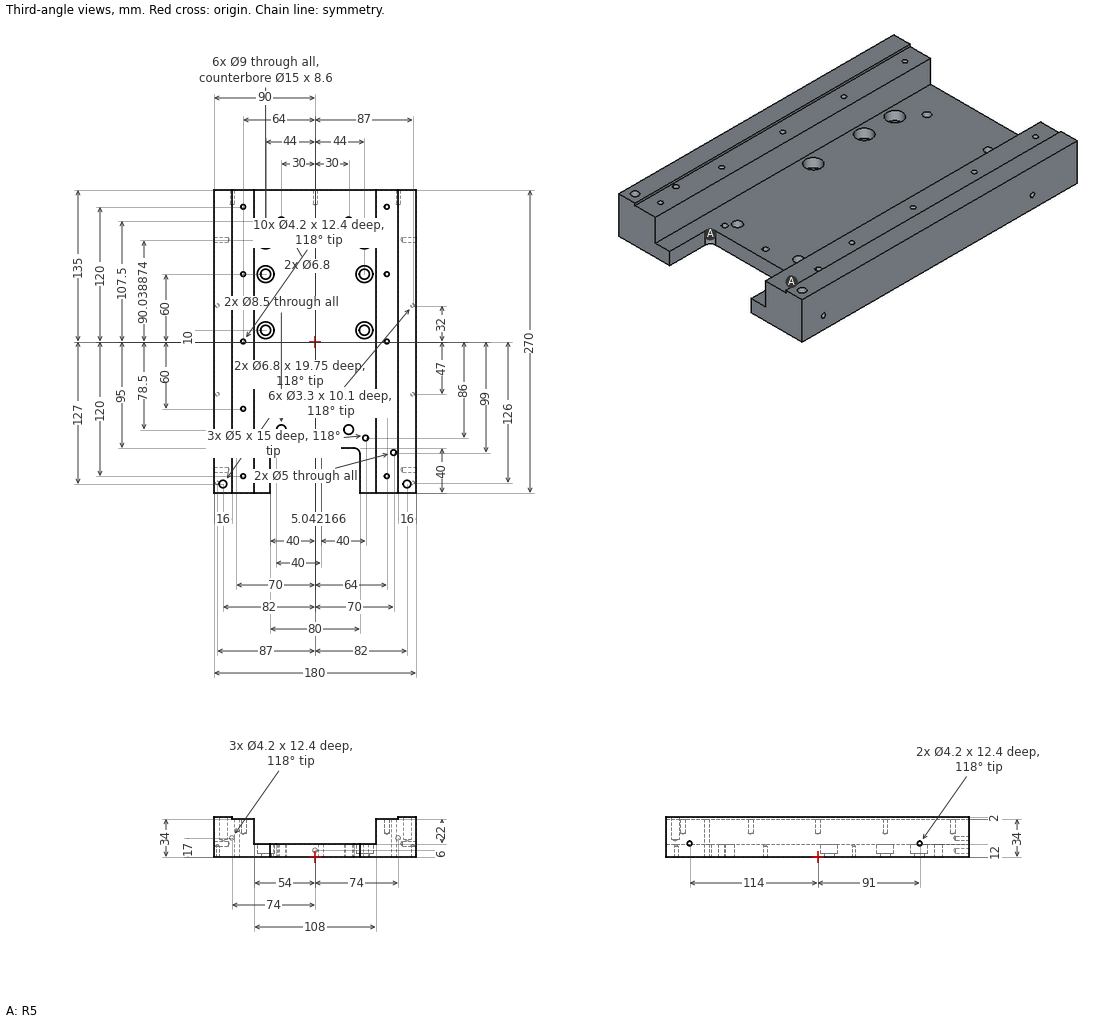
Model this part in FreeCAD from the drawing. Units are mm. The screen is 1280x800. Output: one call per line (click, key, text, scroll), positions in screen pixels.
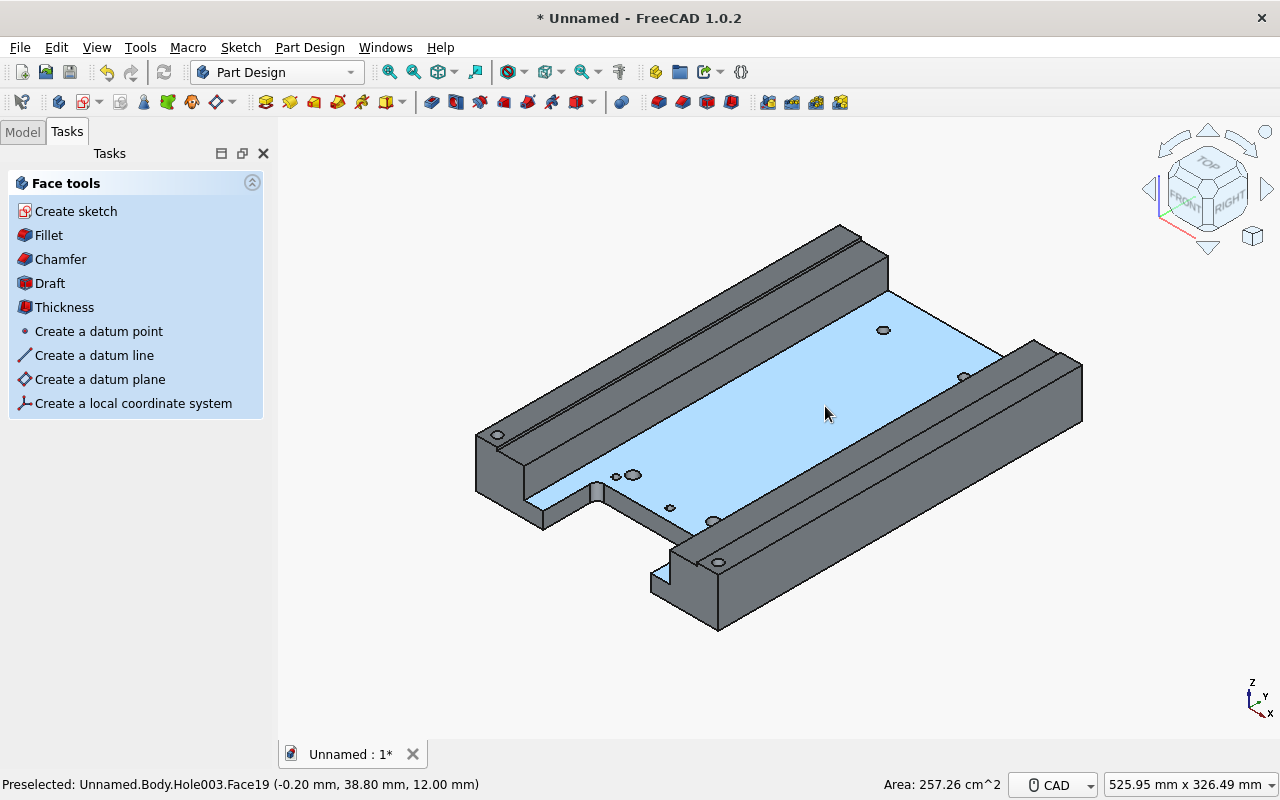
click(84, 102)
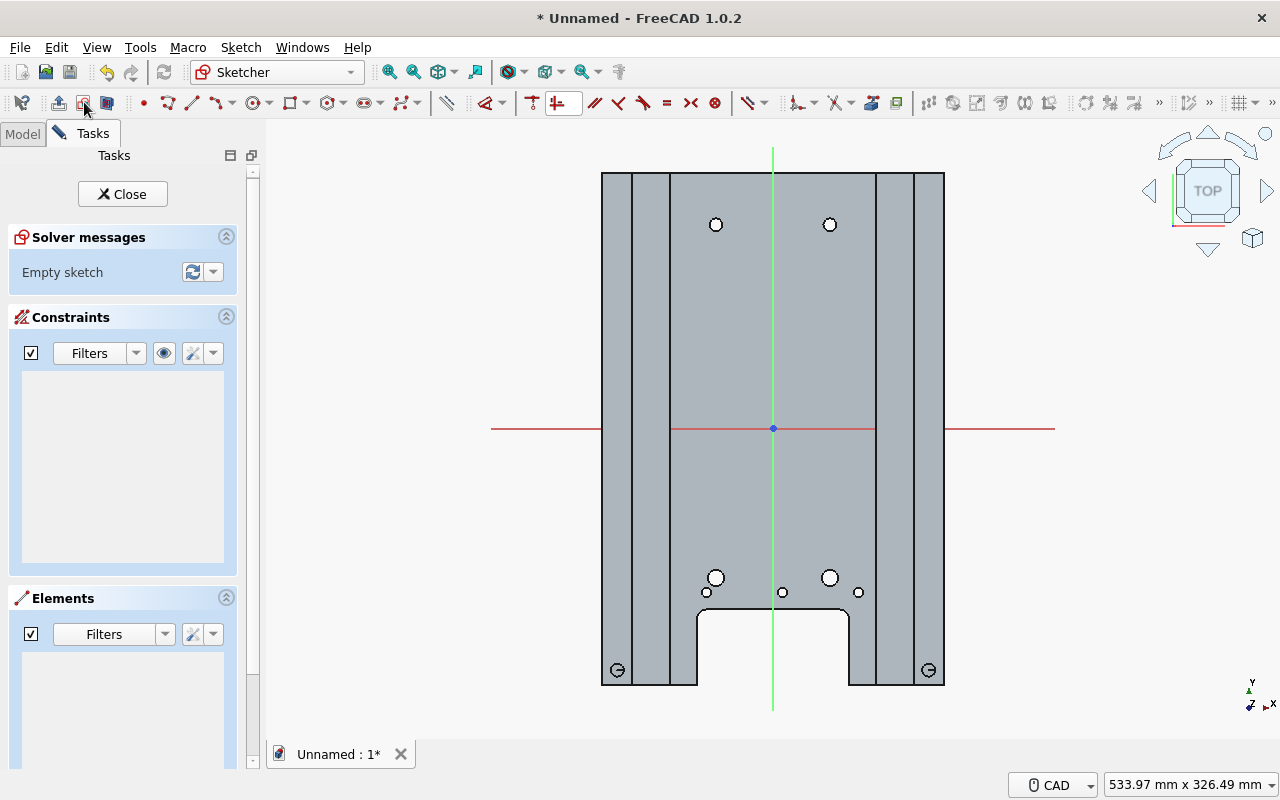
key(q)
key(s)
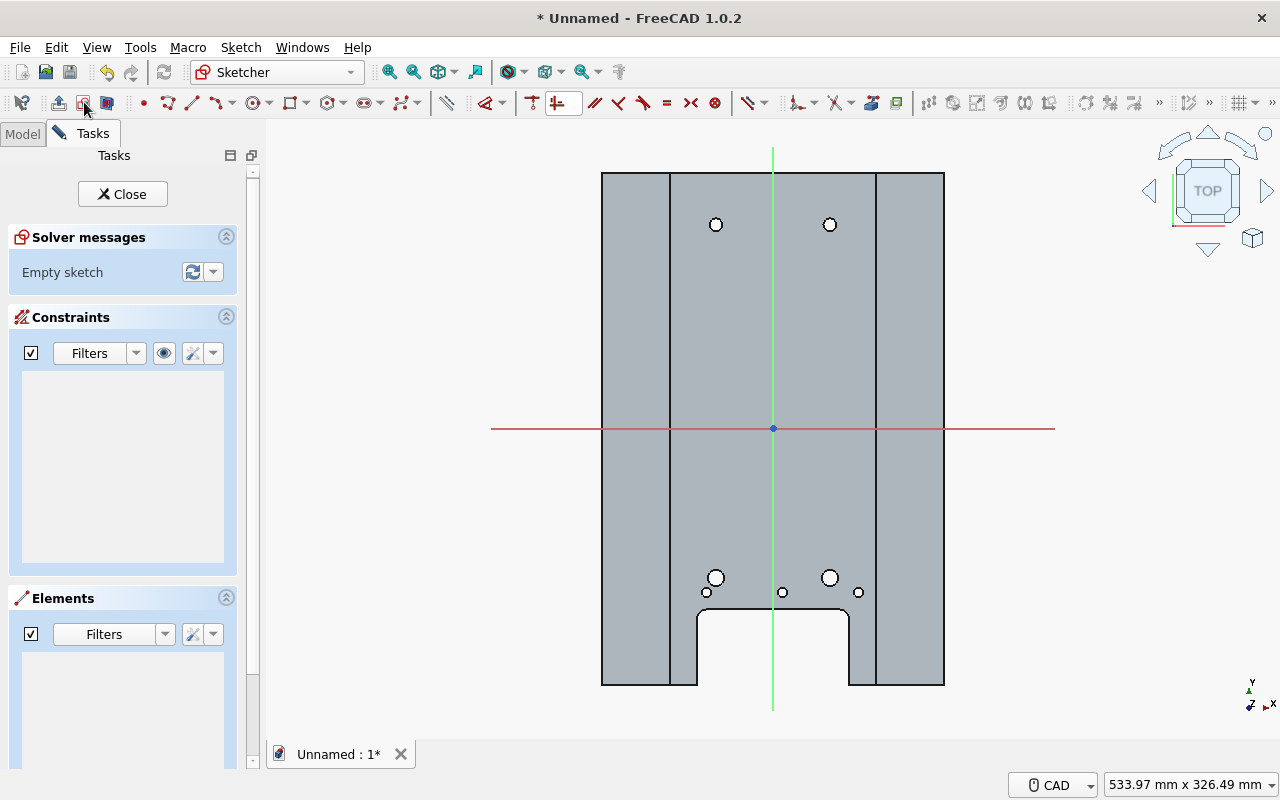
scroll(829, 266, up, 4)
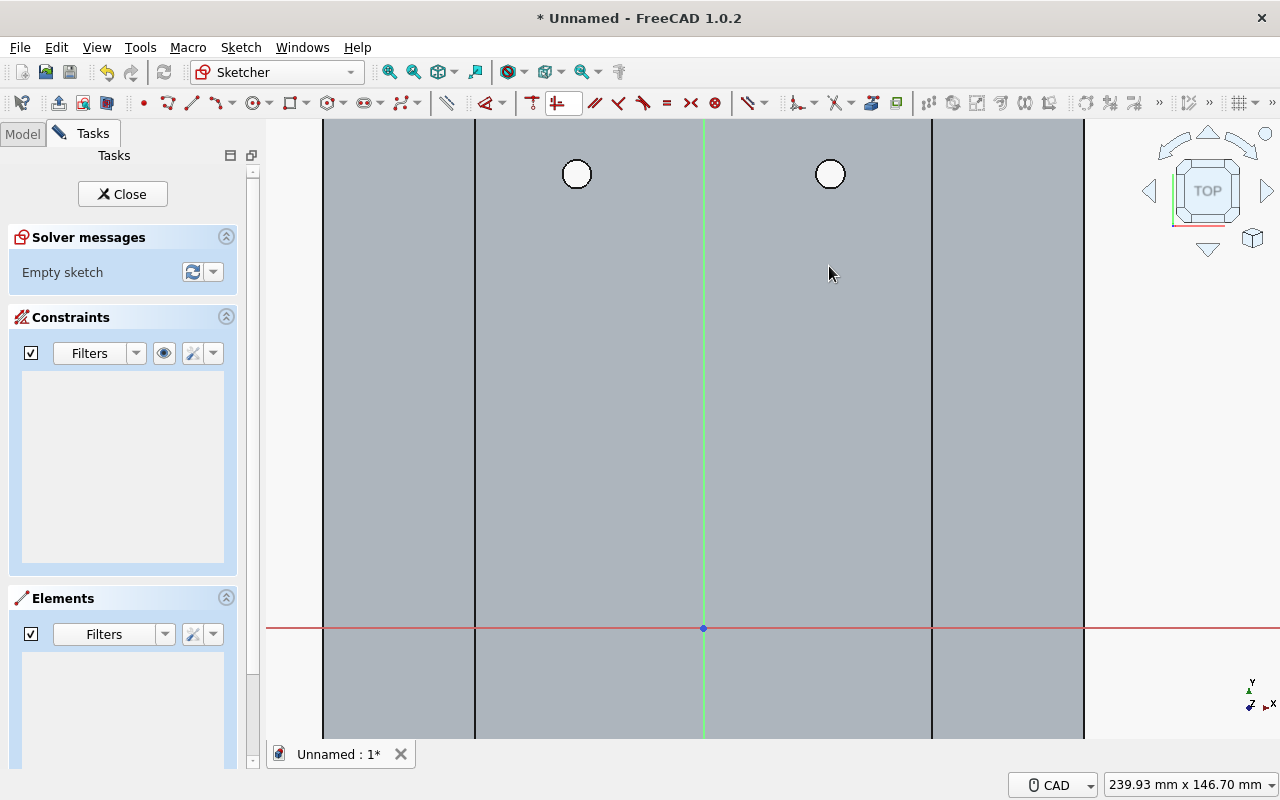
click(254, 104)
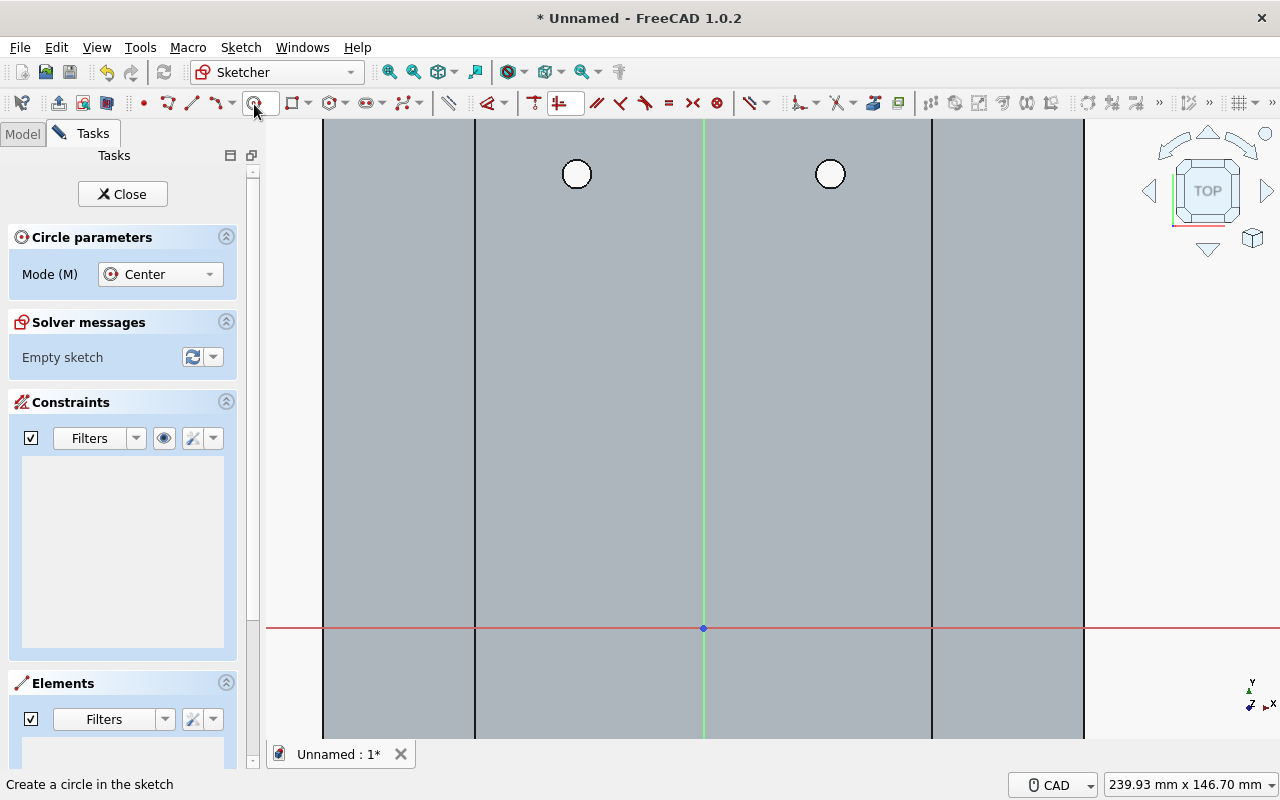
click(518, 248)
move(531, 234)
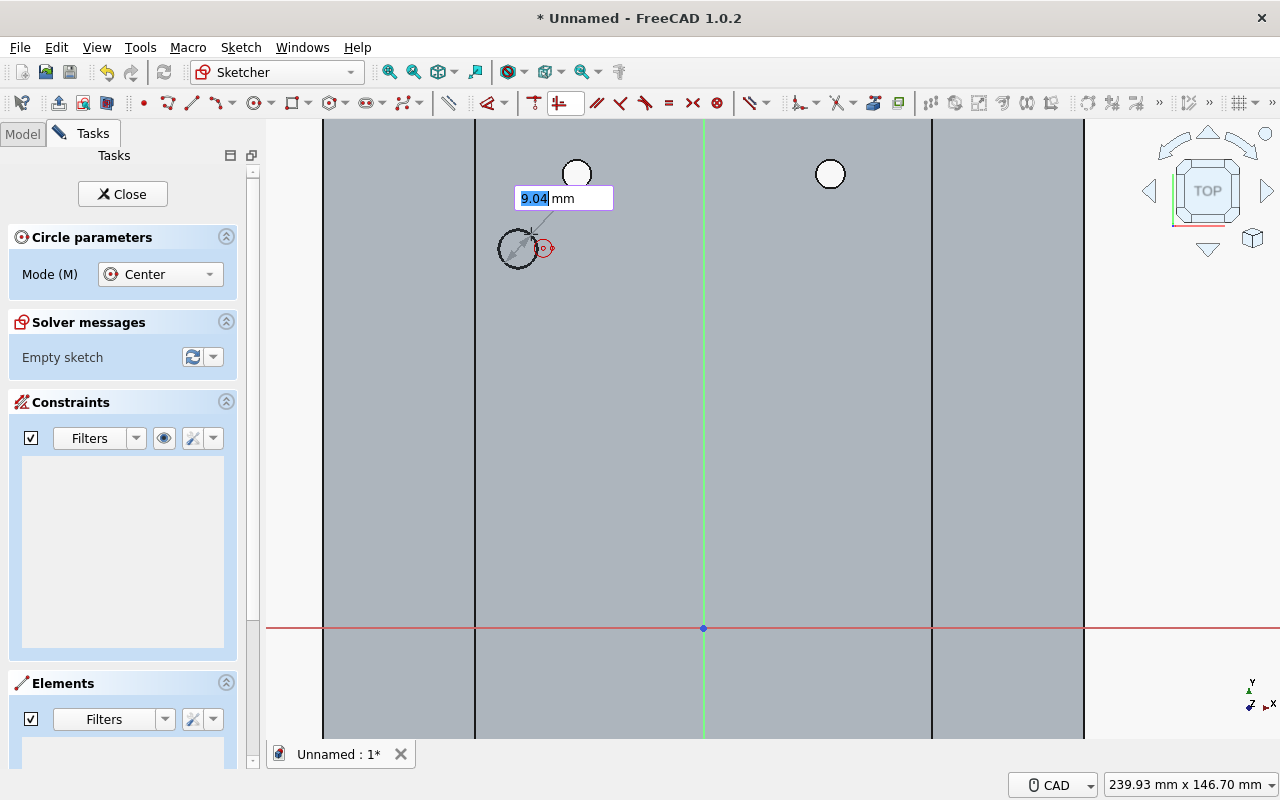
text(9)
key(Return)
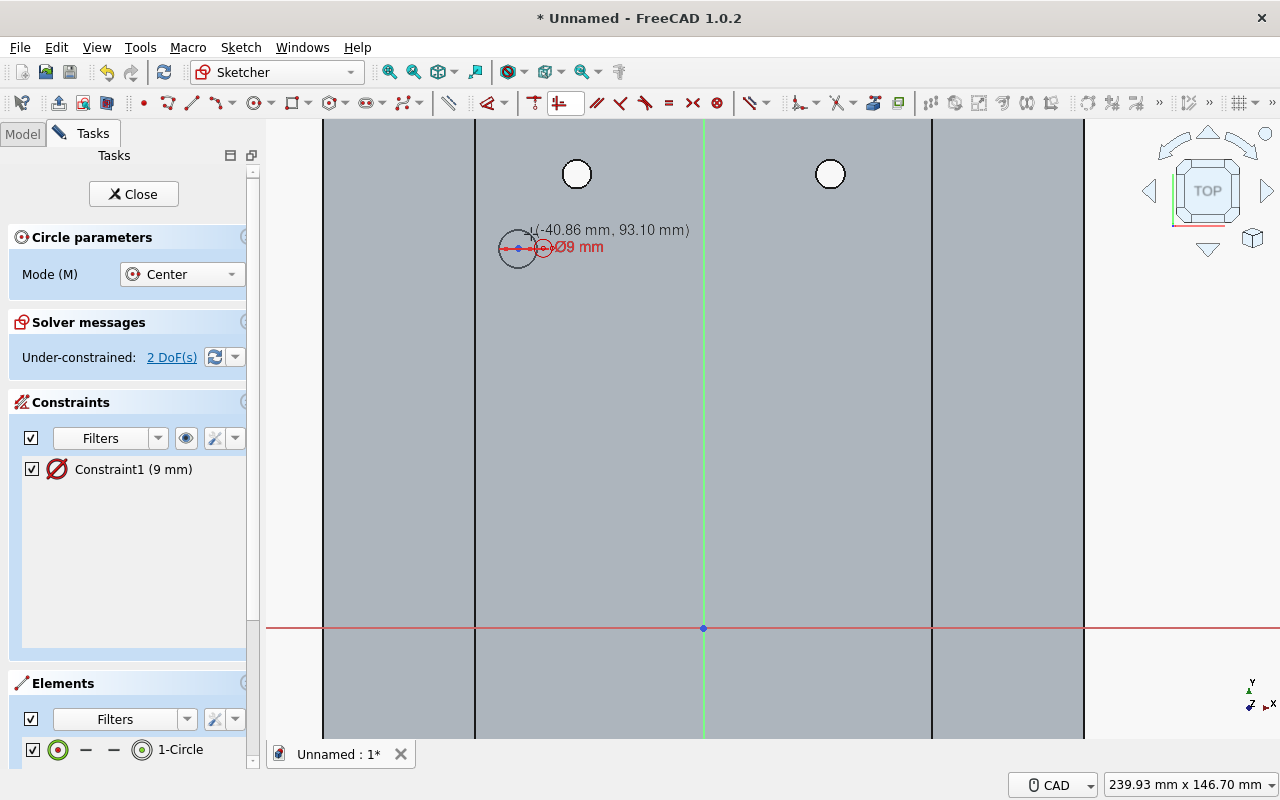
click(518, 586)
move(531, 573)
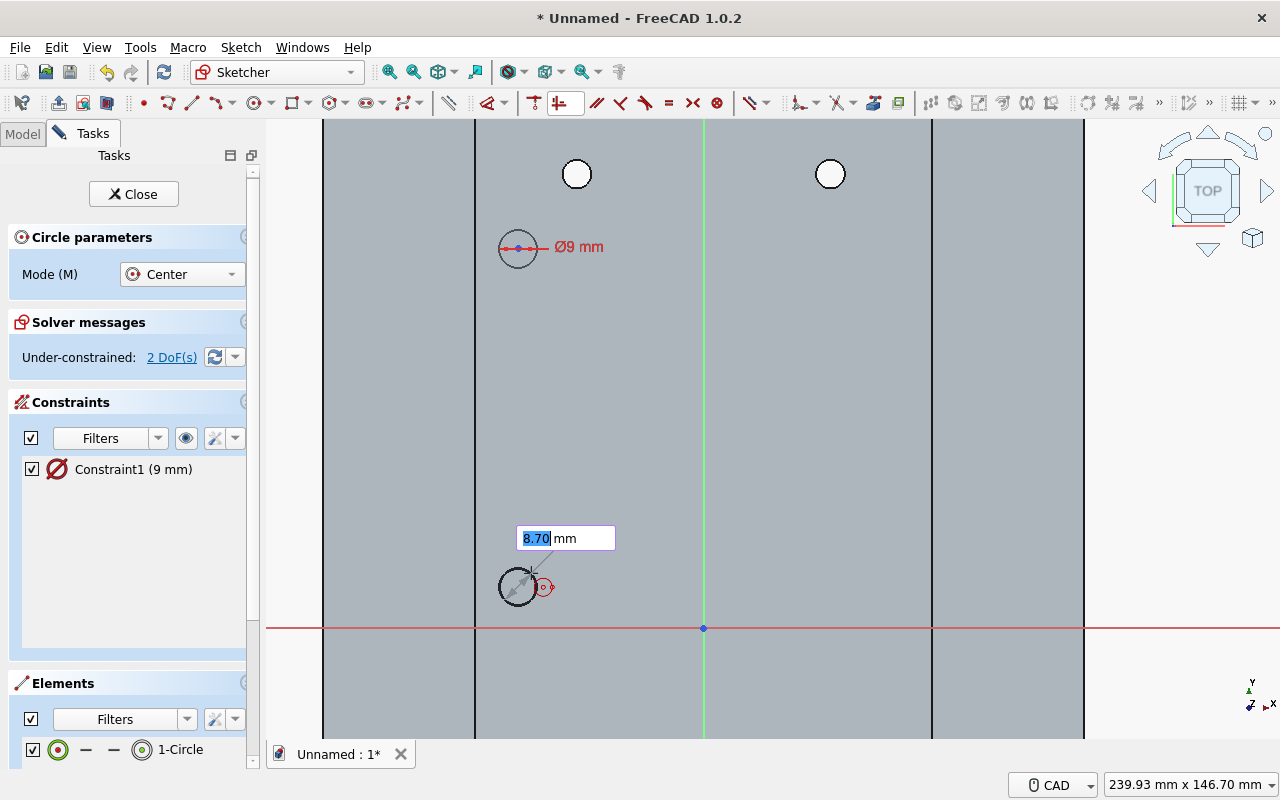
text(9)
key(Return)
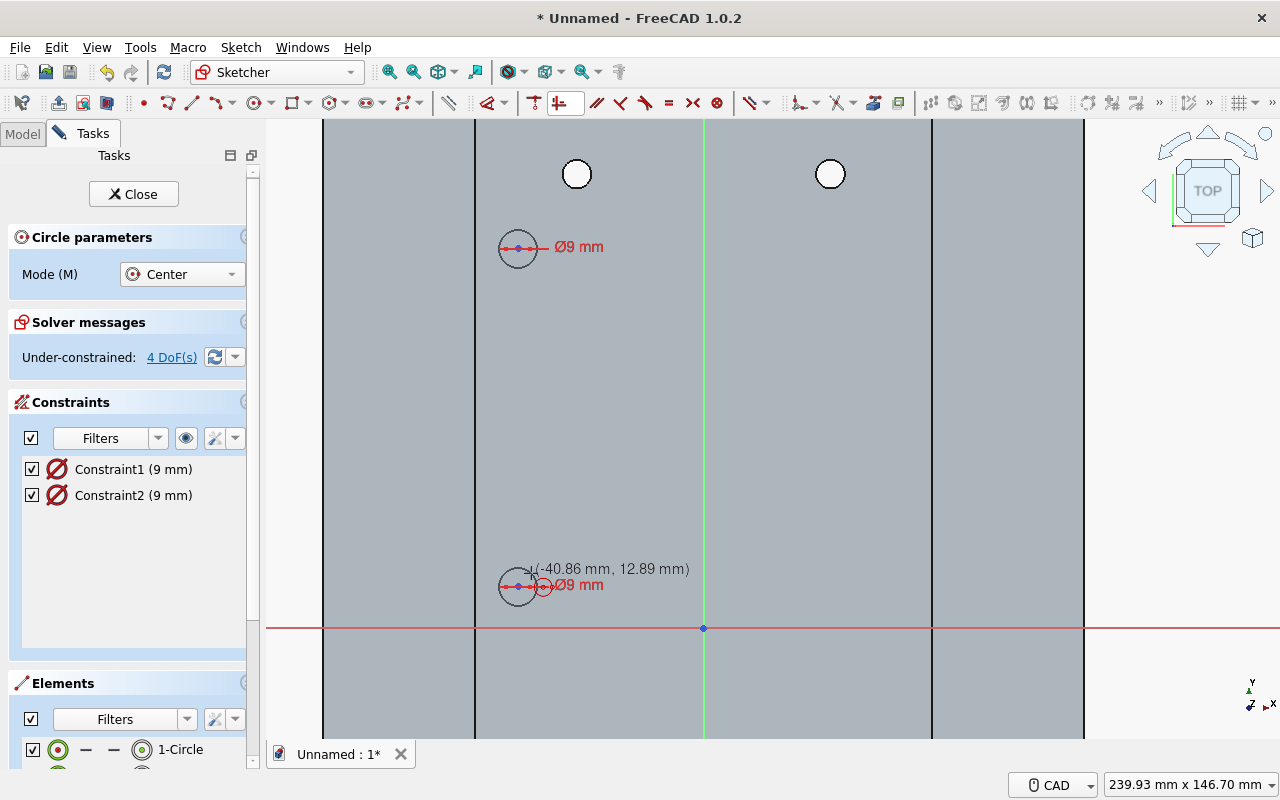
click(518, 375)
move(531, 361)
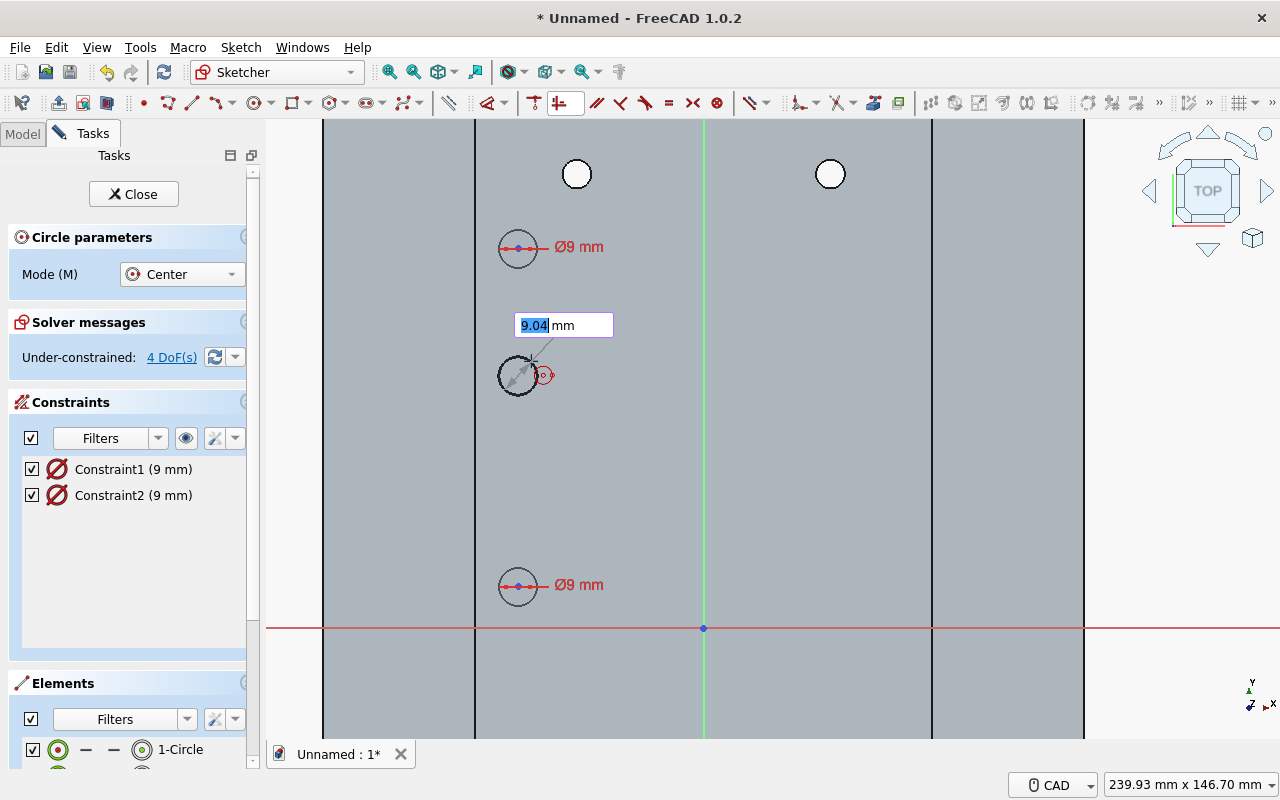
text(9)
key(Return)